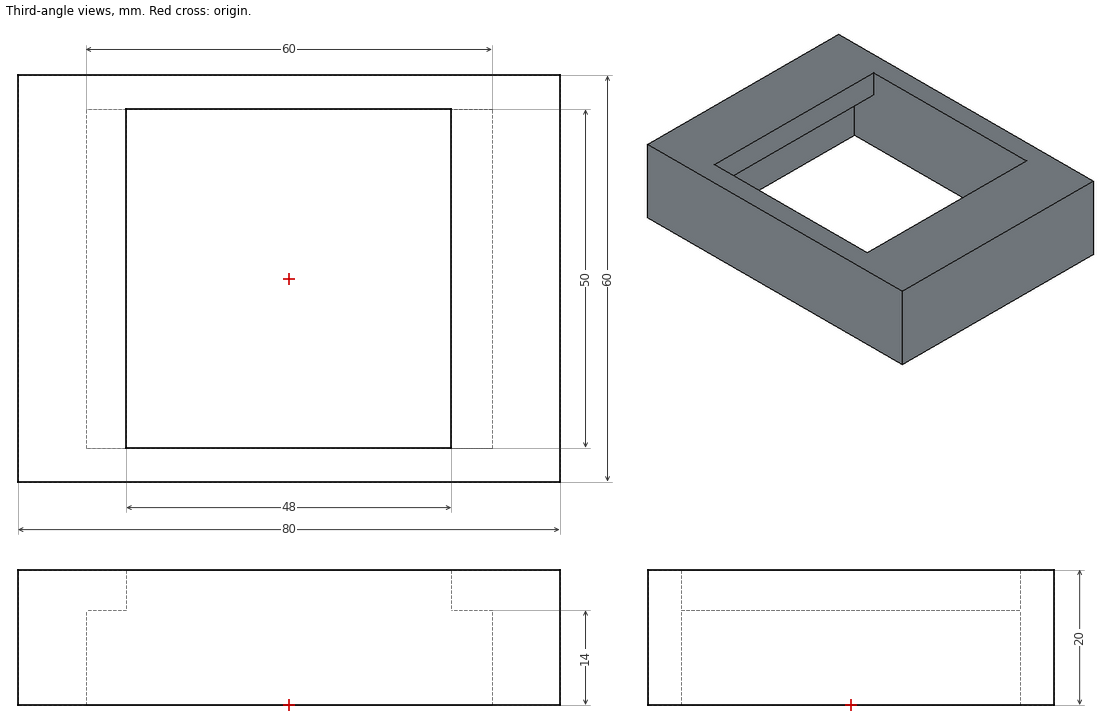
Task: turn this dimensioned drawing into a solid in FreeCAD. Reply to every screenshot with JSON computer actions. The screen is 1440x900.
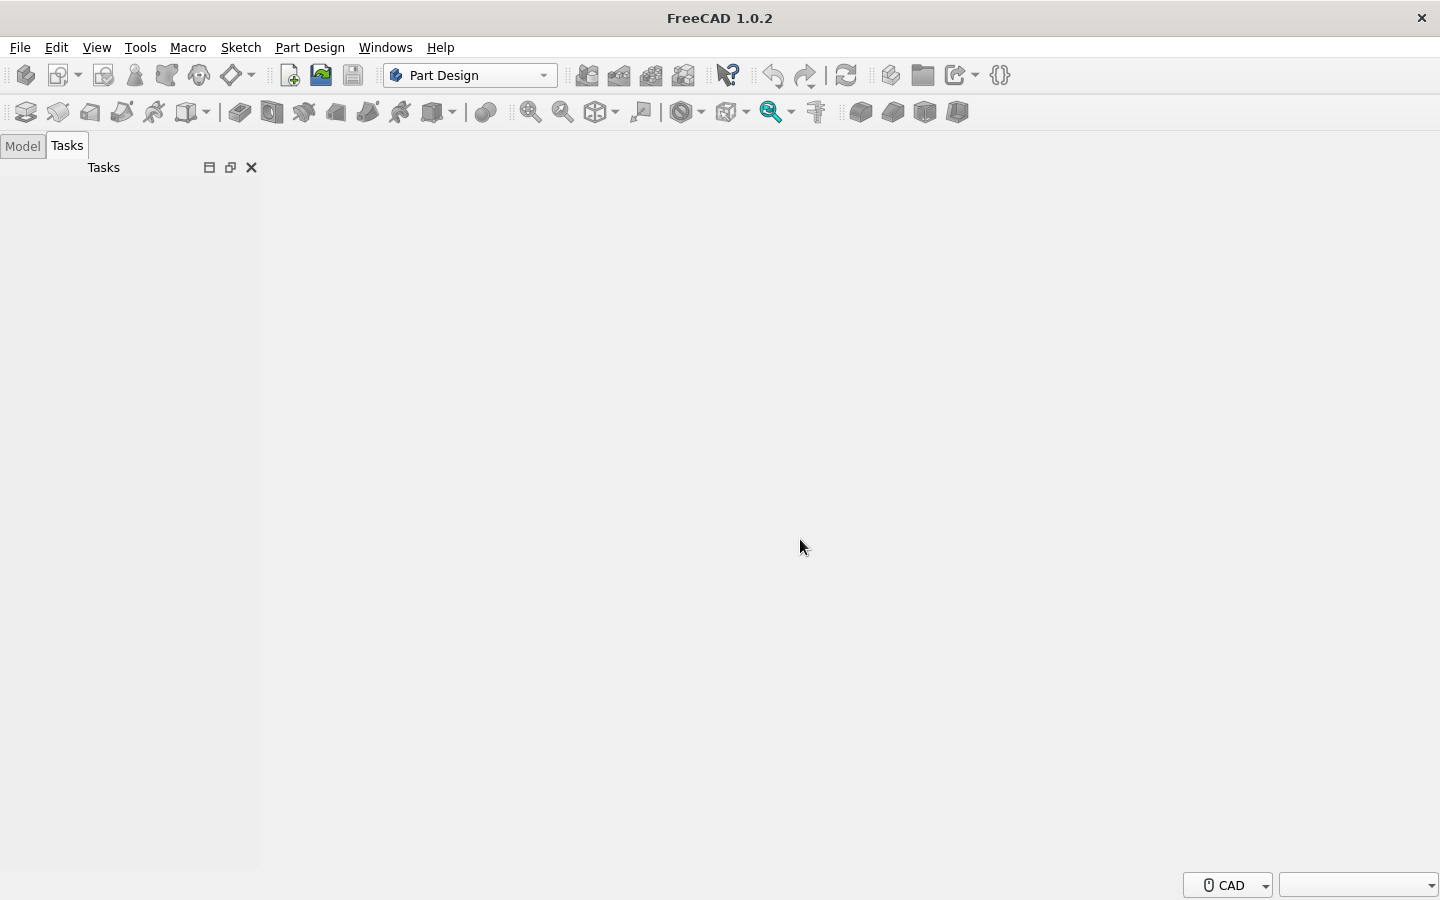
{"action": "key", "text": "ctrl+n"}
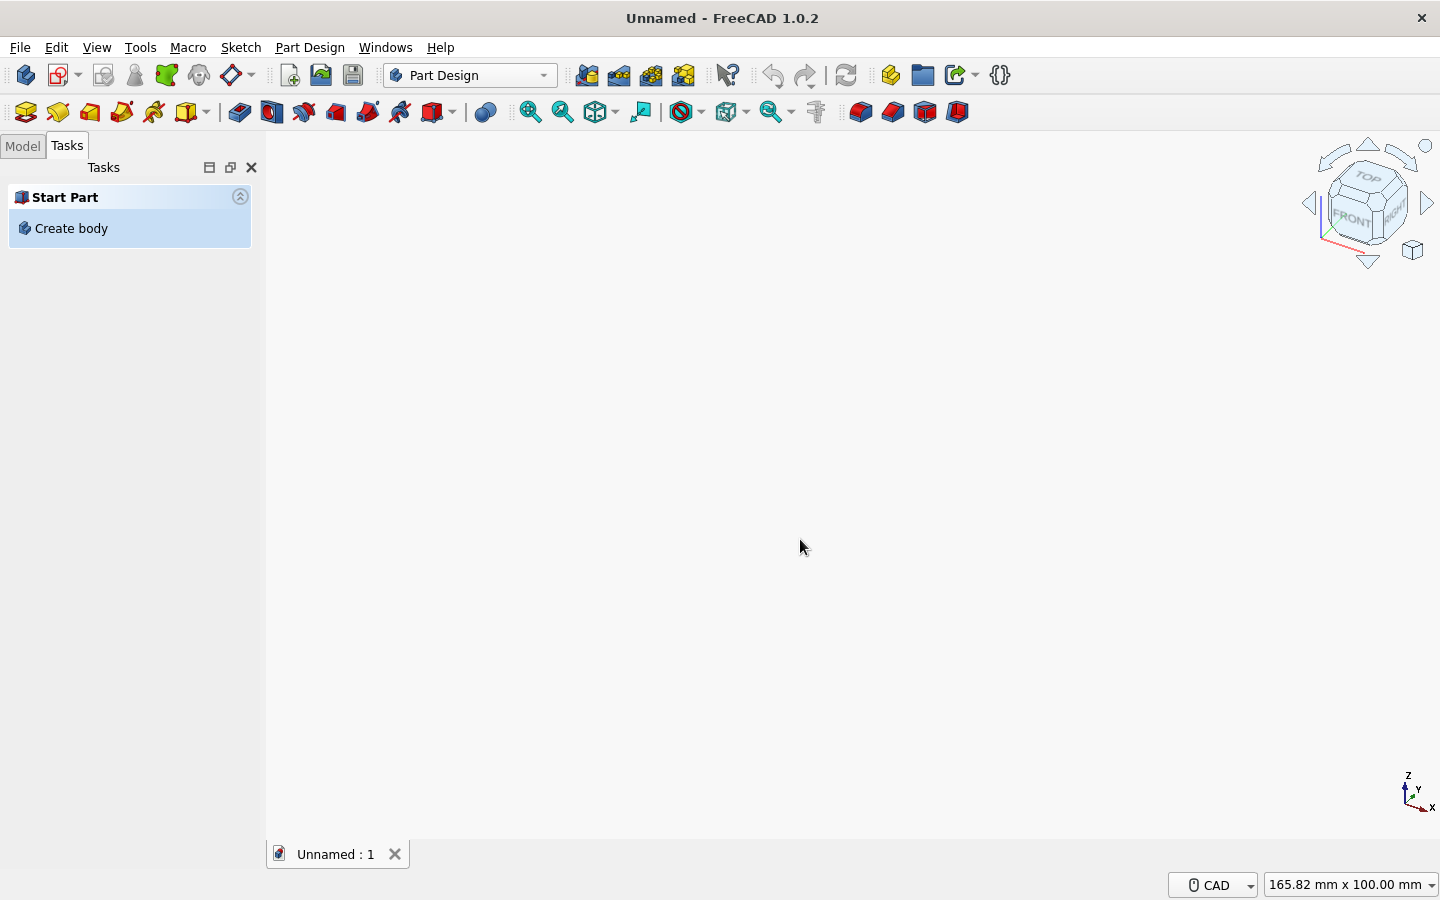
{"action": "left_click", "coordinate": [58, 76]}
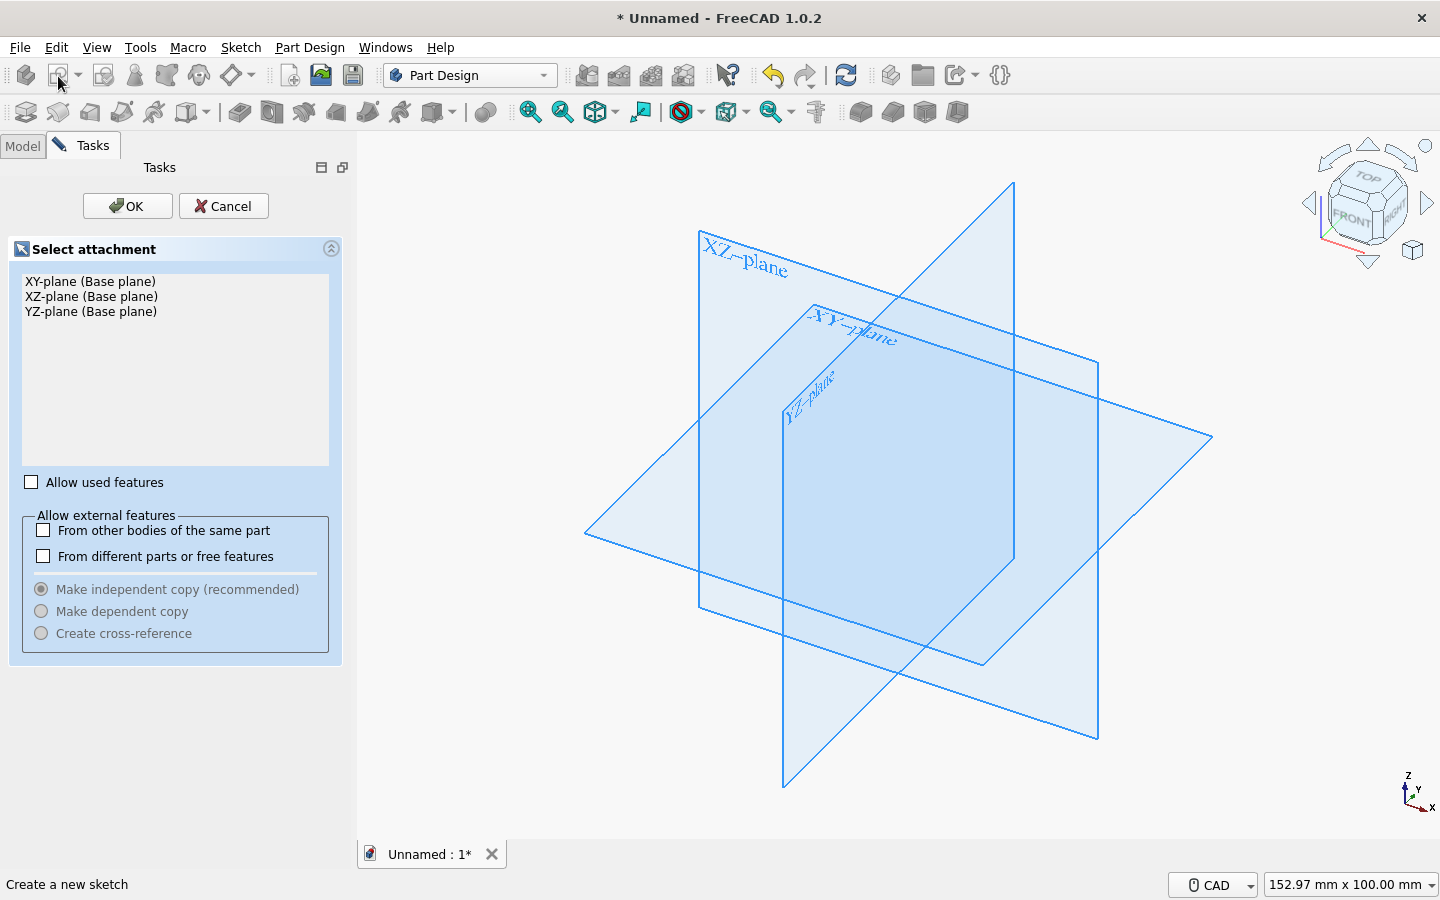
{"action": "left_click", "coordinate": [82, 282]}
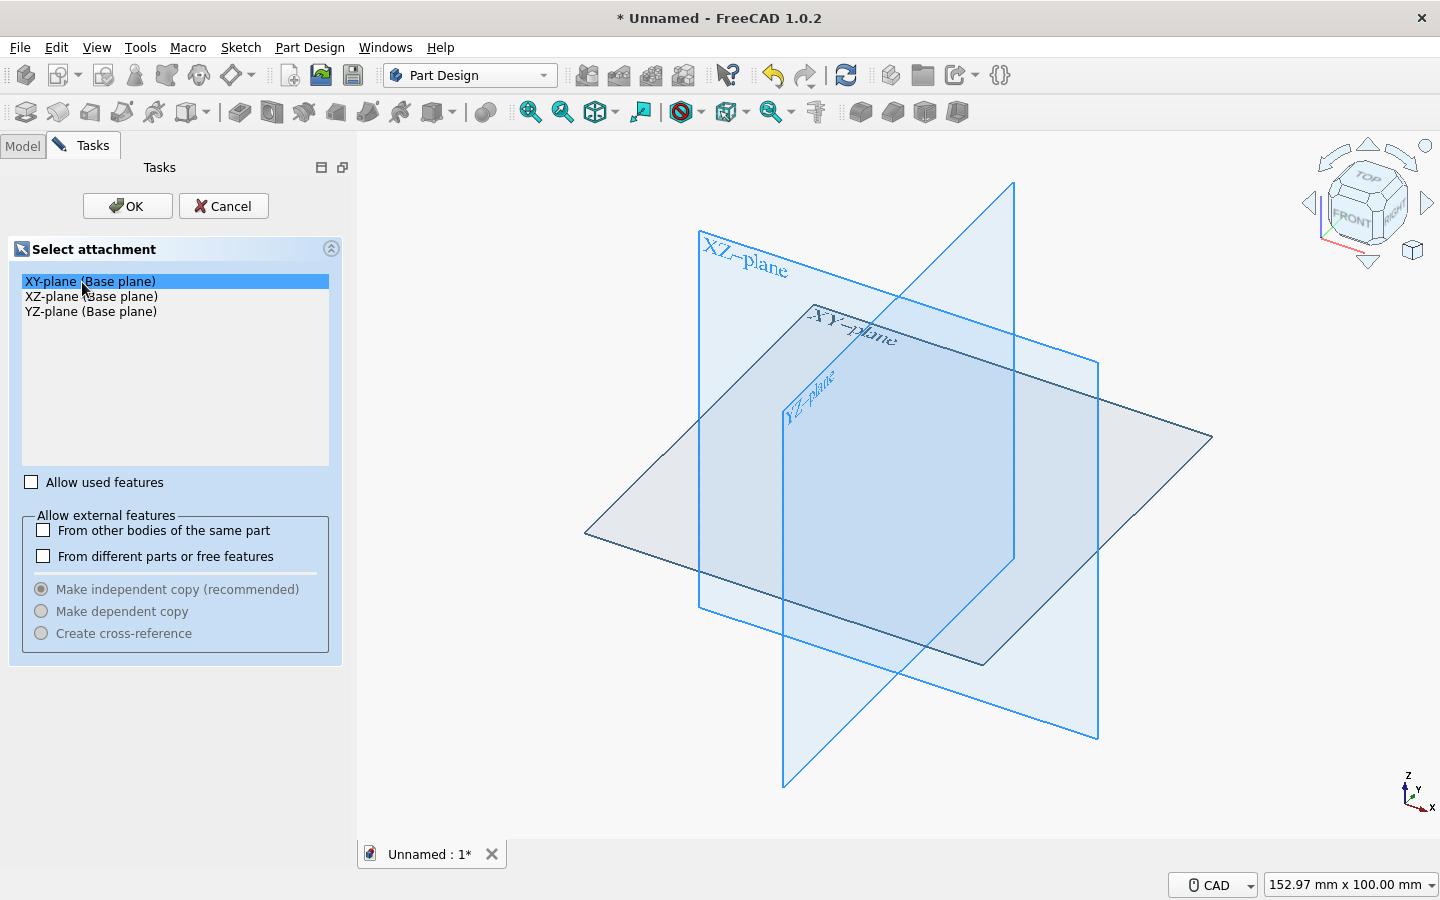
{"action": "left_click", "coordinate": [128, 206]}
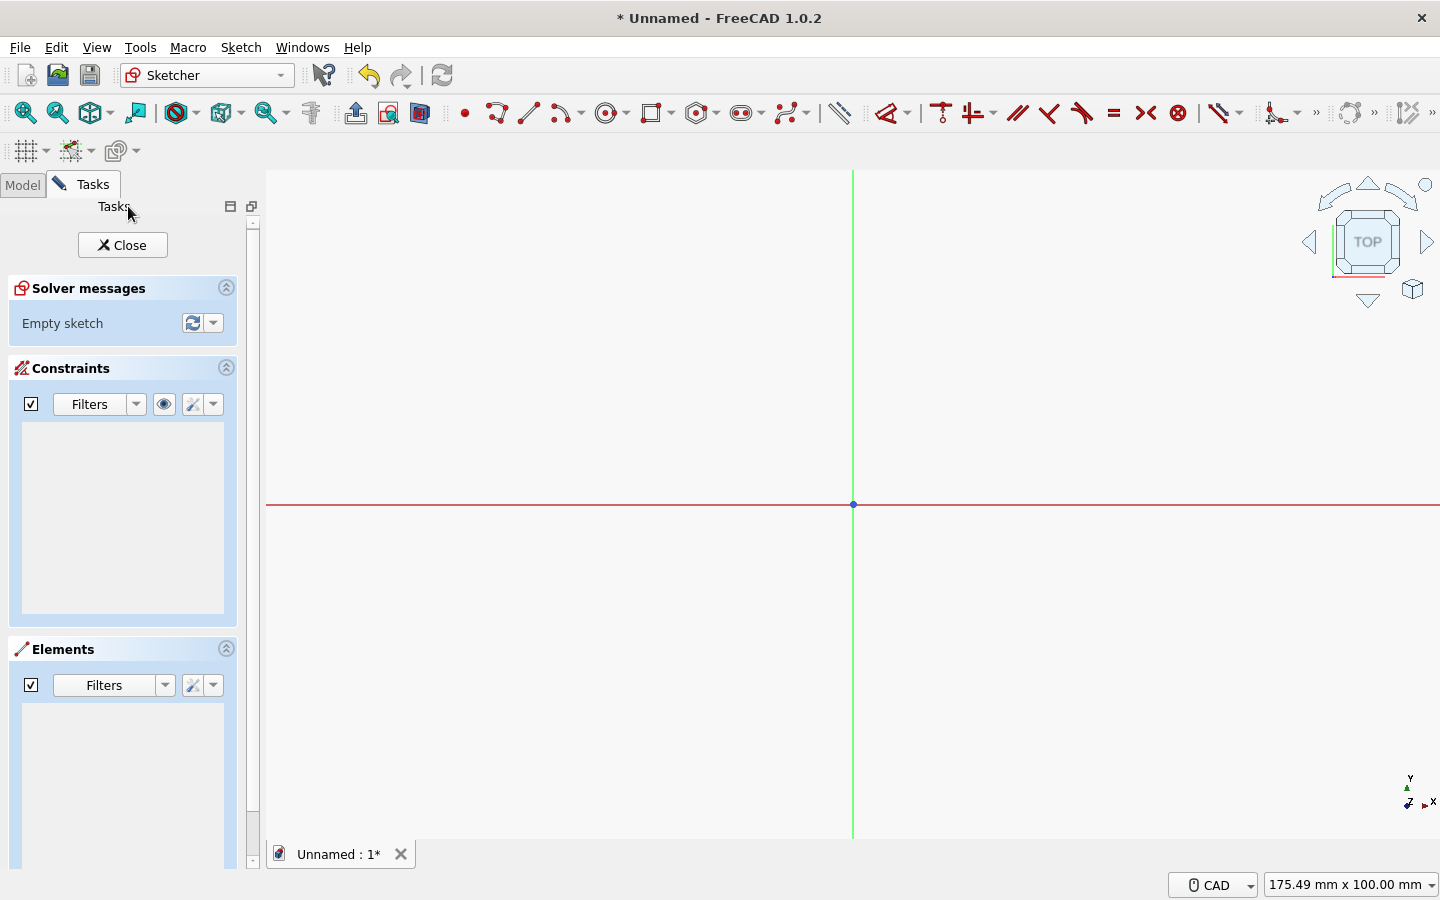
{"action": "key", "text": "g v"}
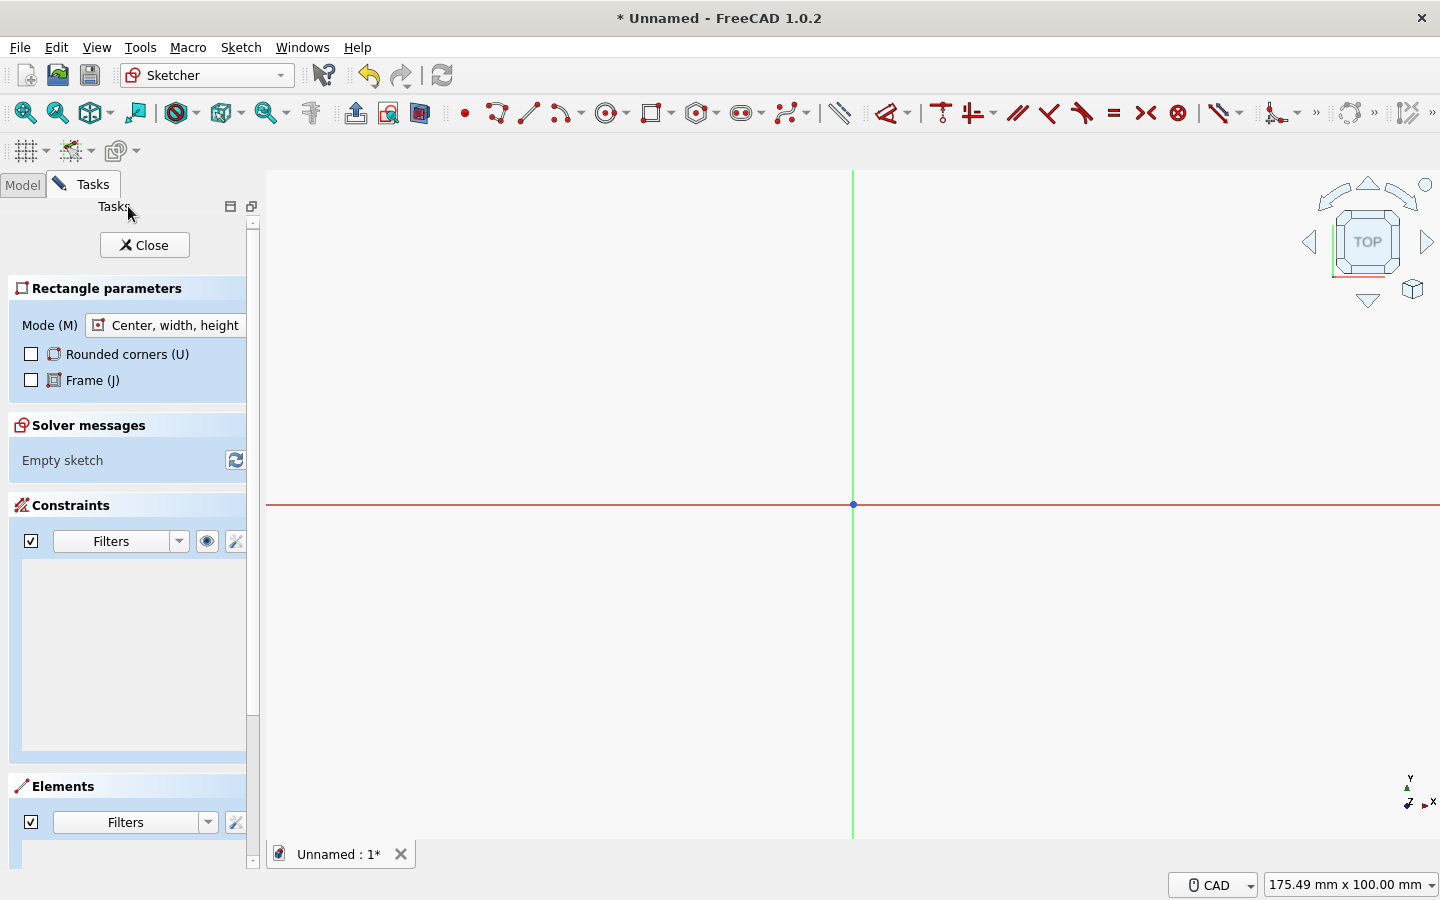
{"action": "left_click", "coordinate": [853, 504]}
{"action": "mouse_move", "coordinate": [1121, 304]}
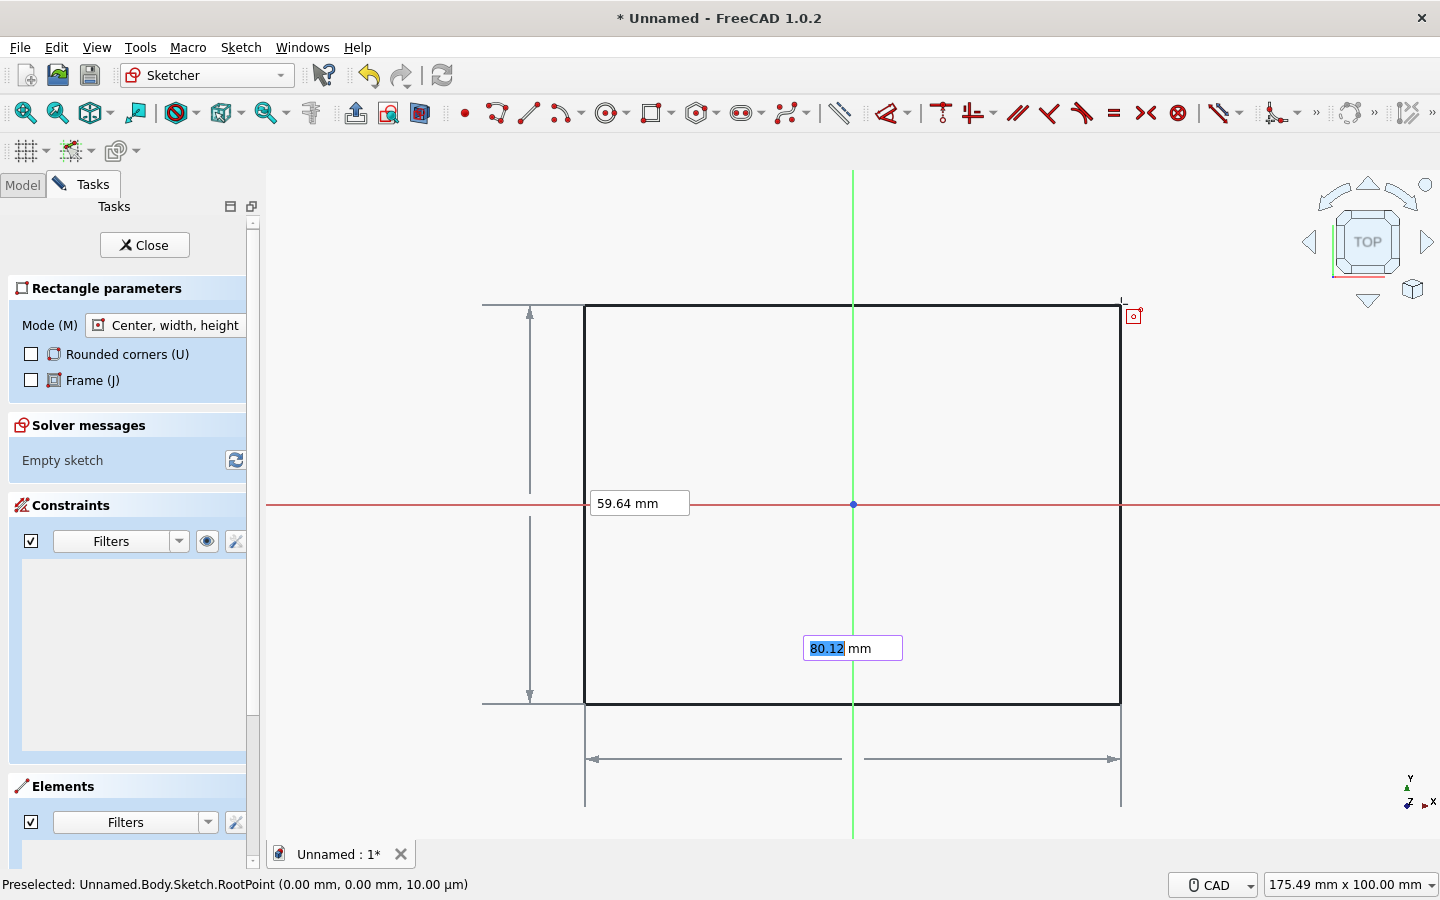
{"action": "type", "text": "80"}
{"action": "key", "text": "Tab"}
{"action": "type", "text": "60"}
{"action": "key", "text": "Return"}
{"action": "key", "text": "Escape"}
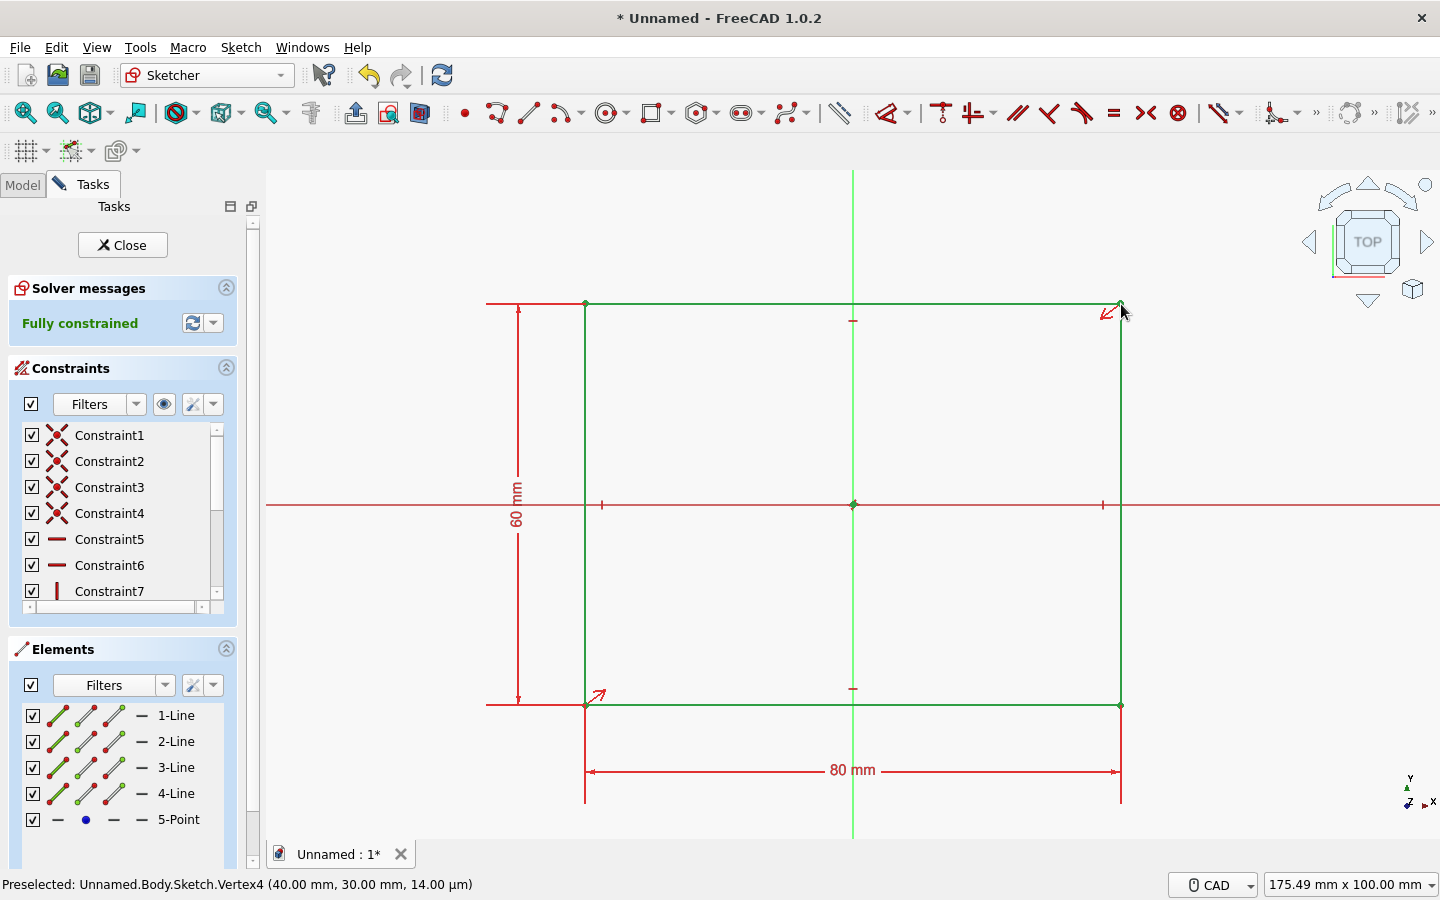
{"action": "left_click", "coordinate": [123, 245]}